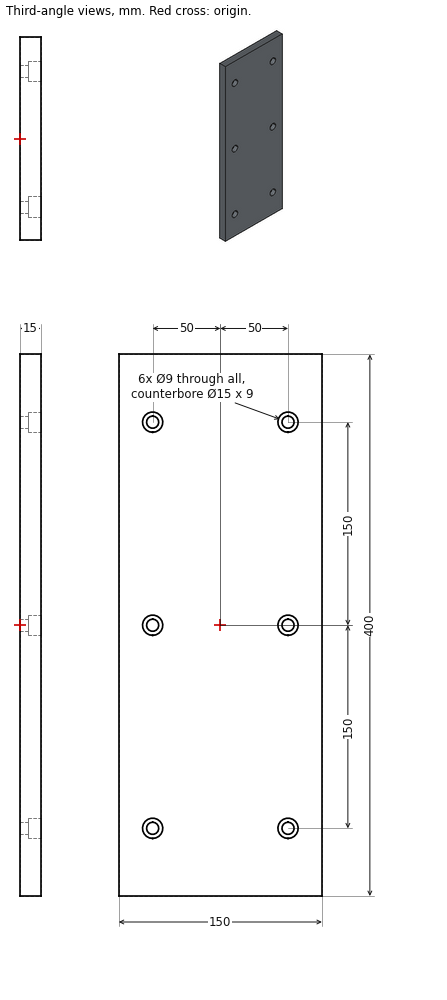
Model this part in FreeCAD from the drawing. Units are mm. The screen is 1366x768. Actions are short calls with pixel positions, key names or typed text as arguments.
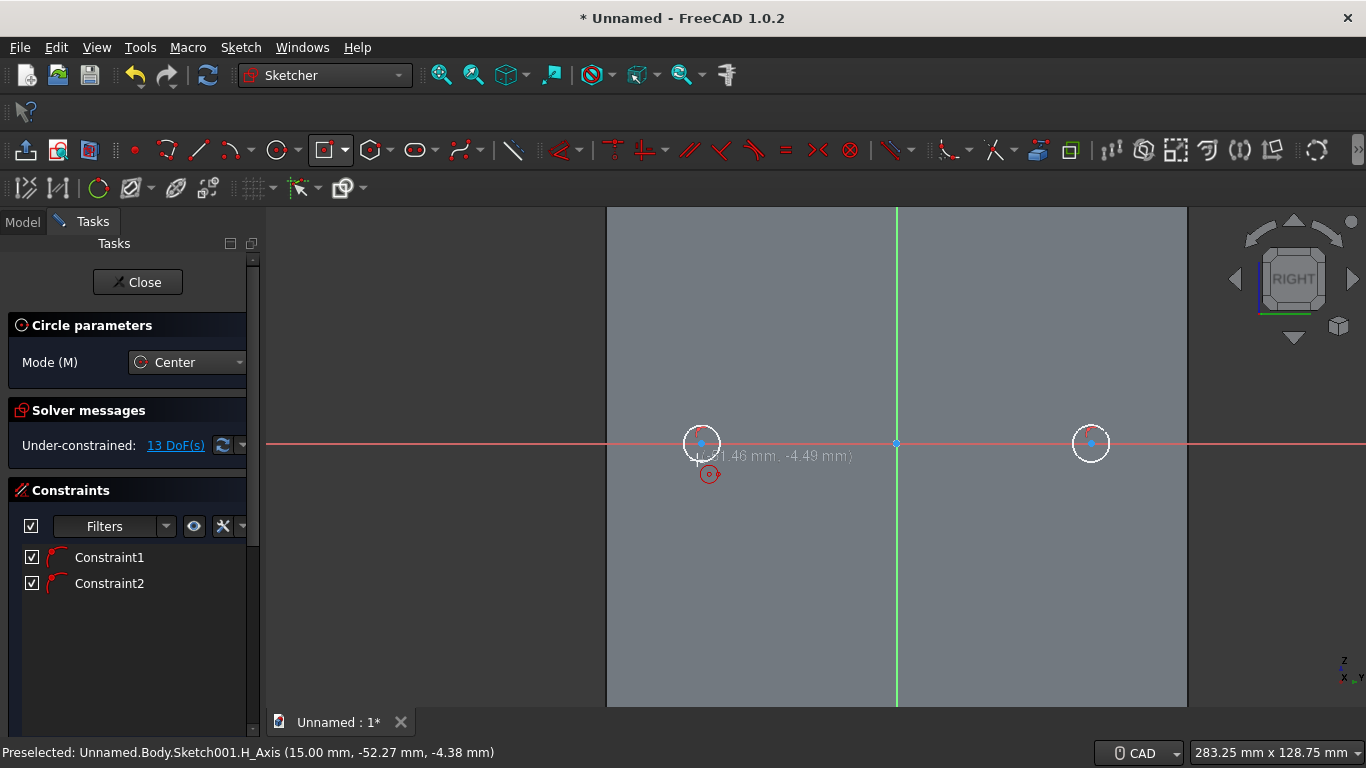
scroll(699, 461, down, 7)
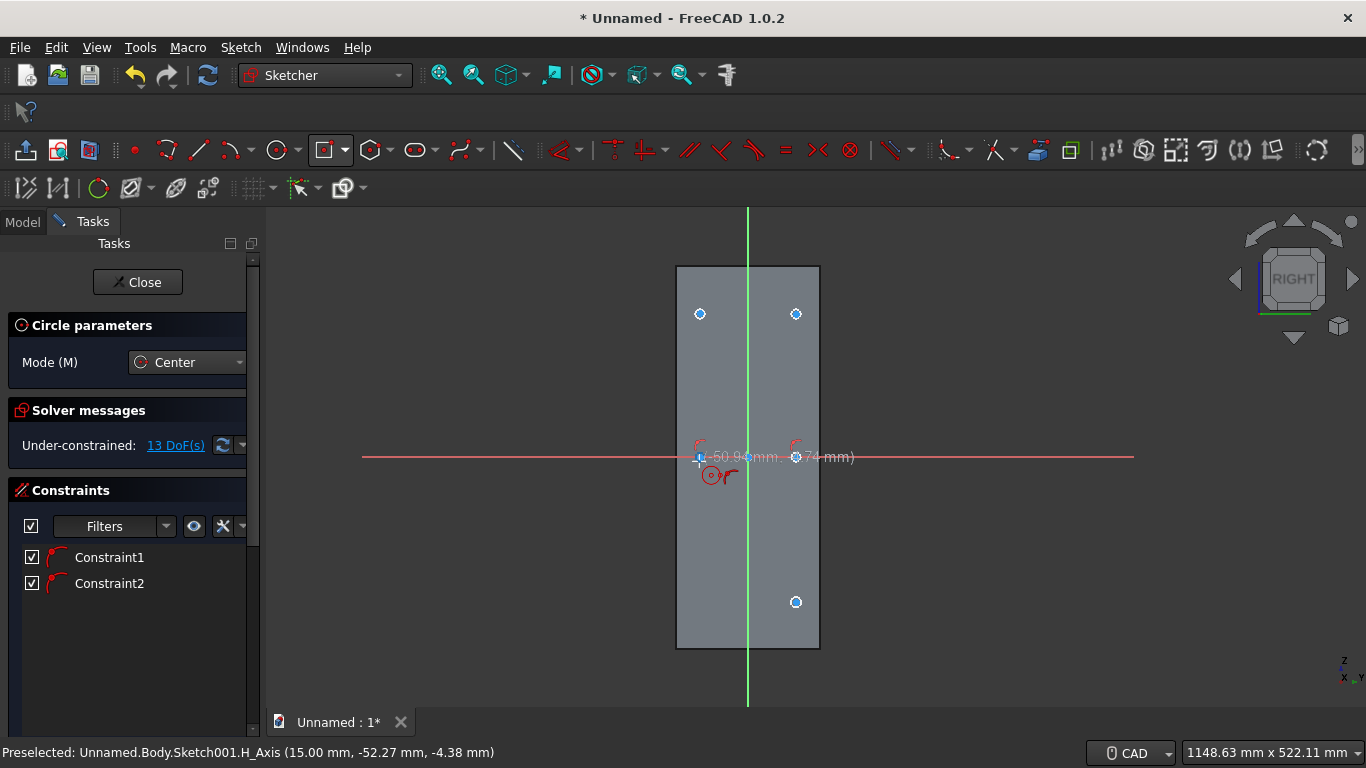
scroll(700, 601, up, 9)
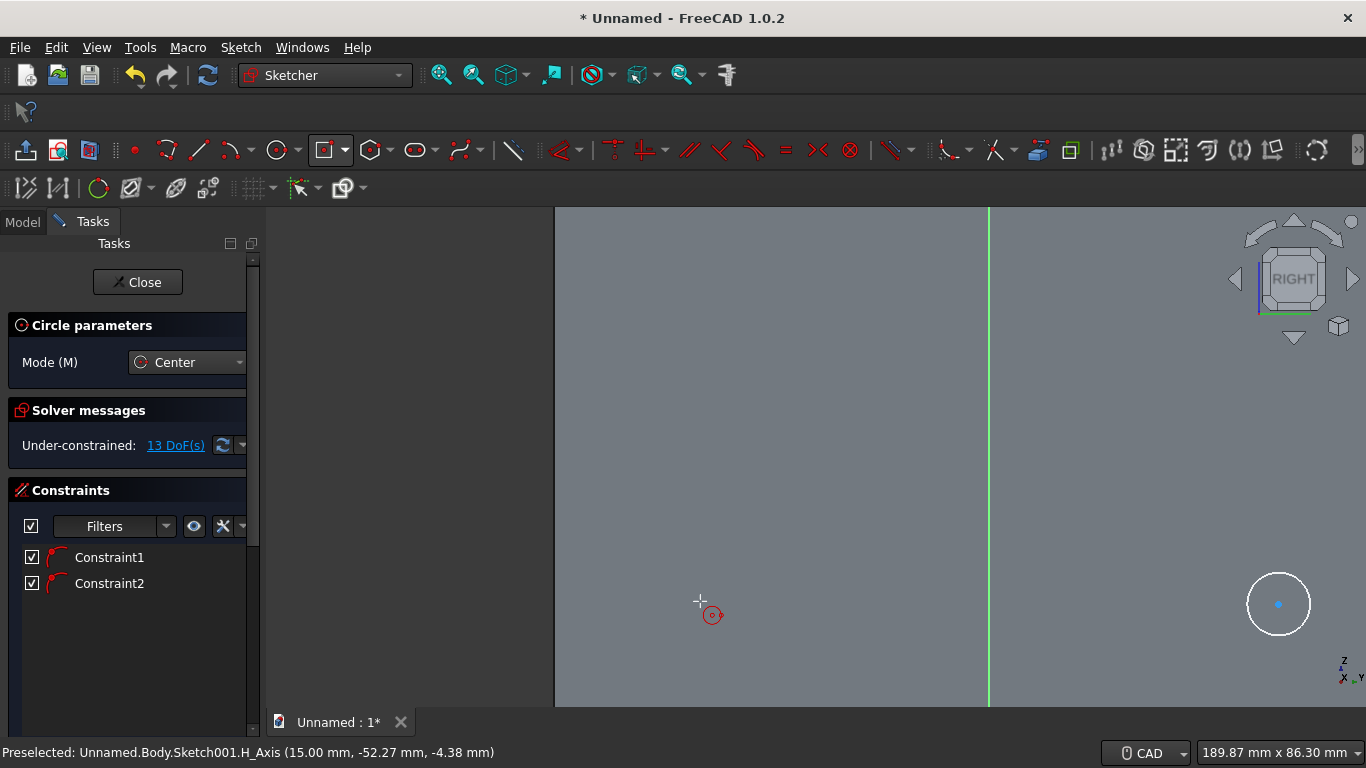
scroll(700, 602, down, 9)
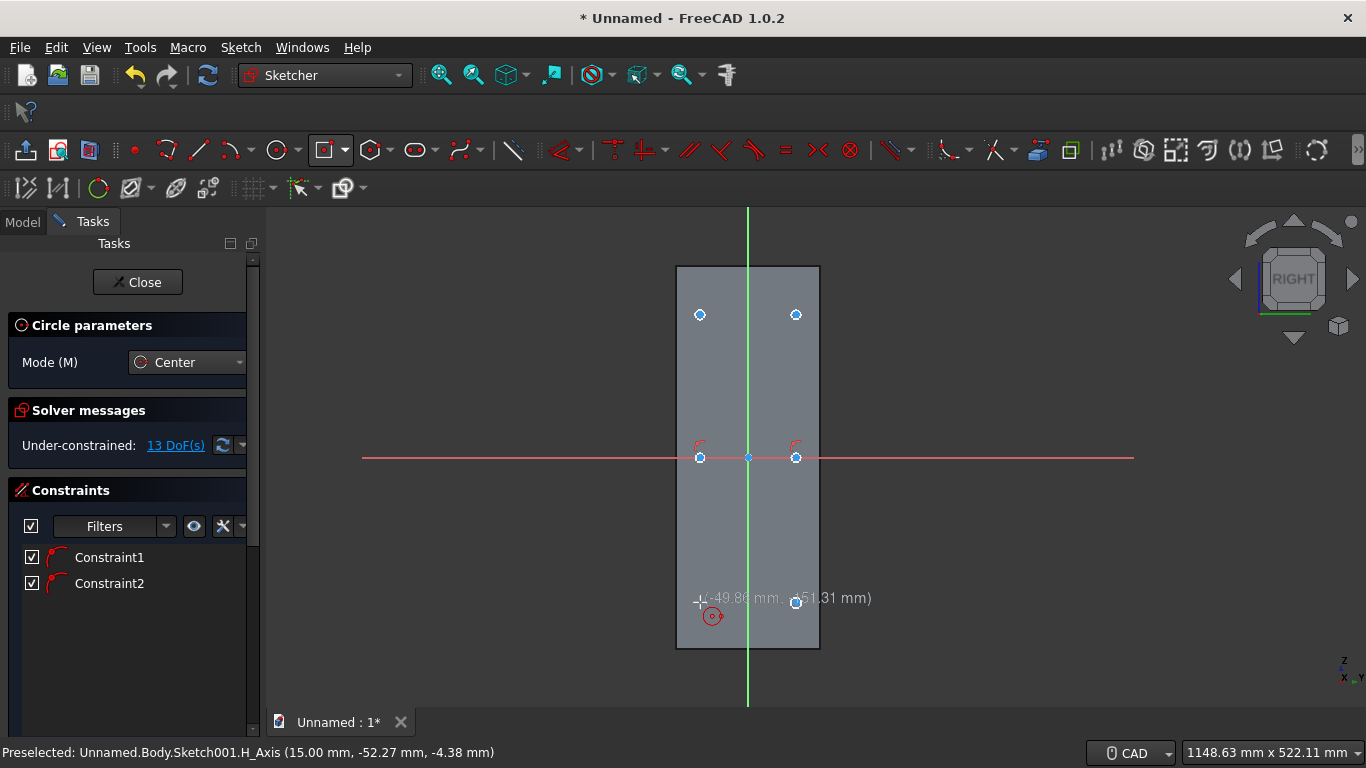
click(700, 602)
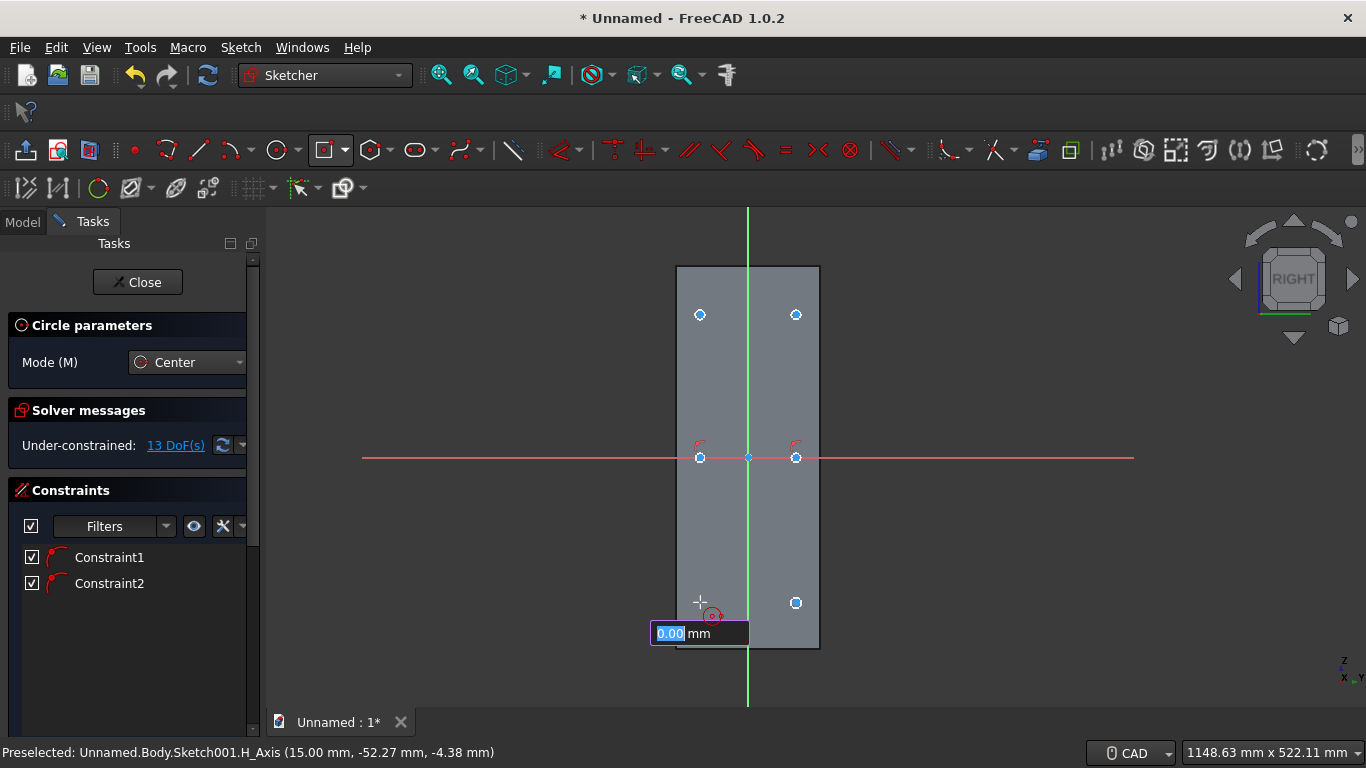
scroll(703, 599, up, 7)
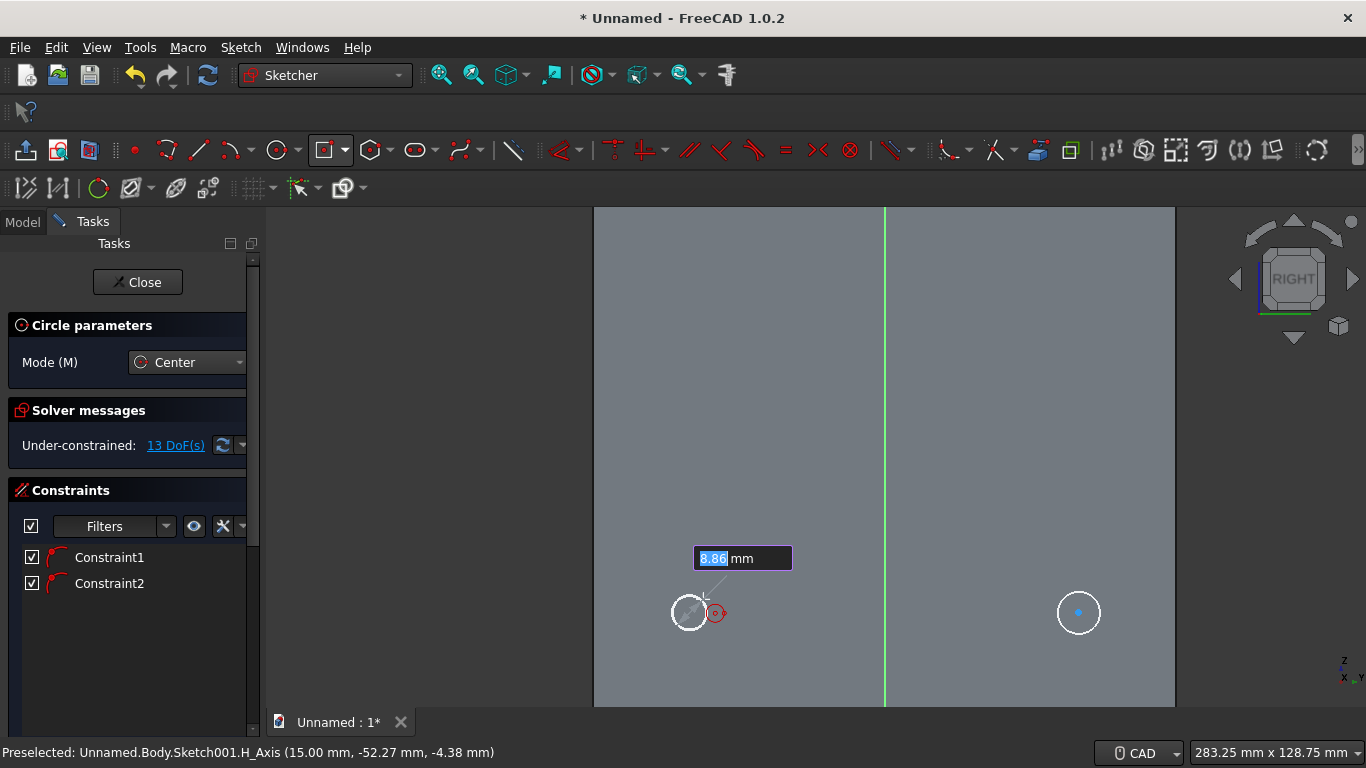
click(703, 595)
key(Escape)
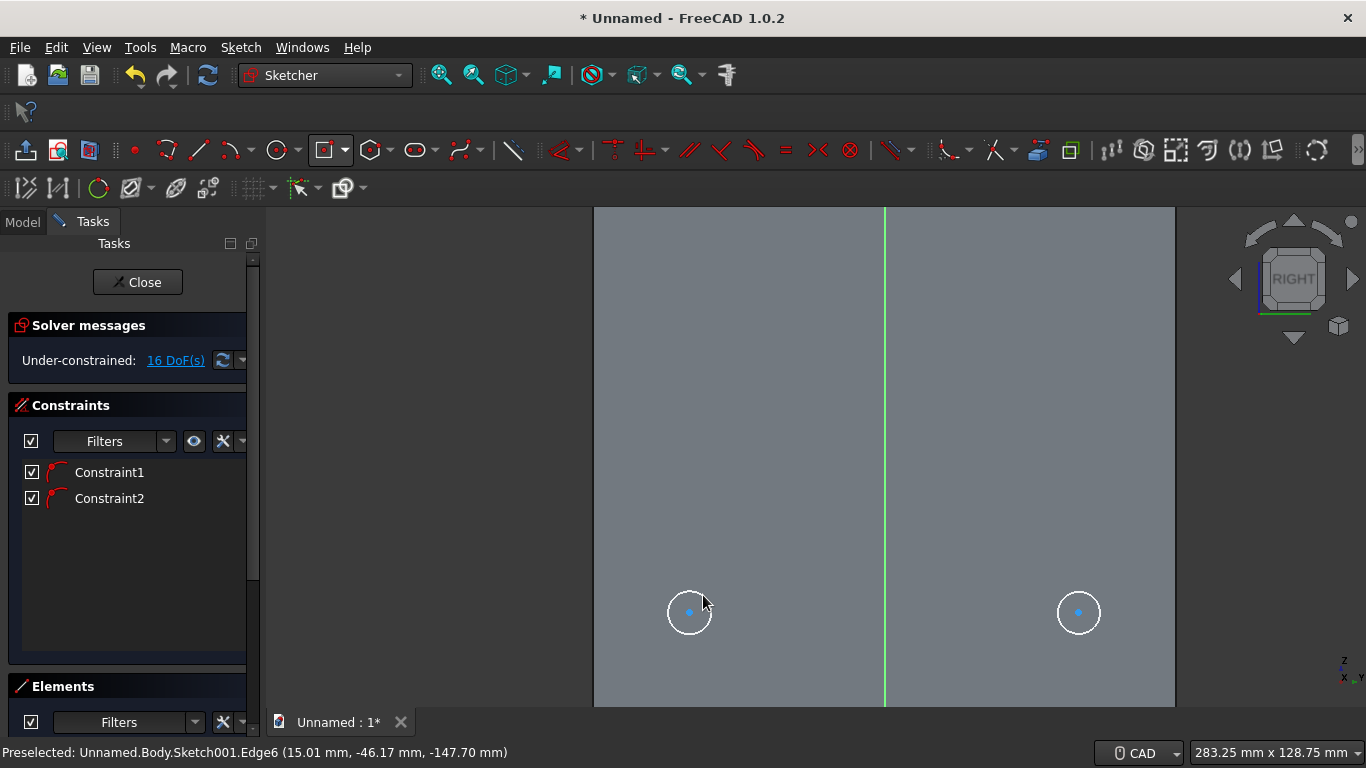
scroll(703, 599, down, 7)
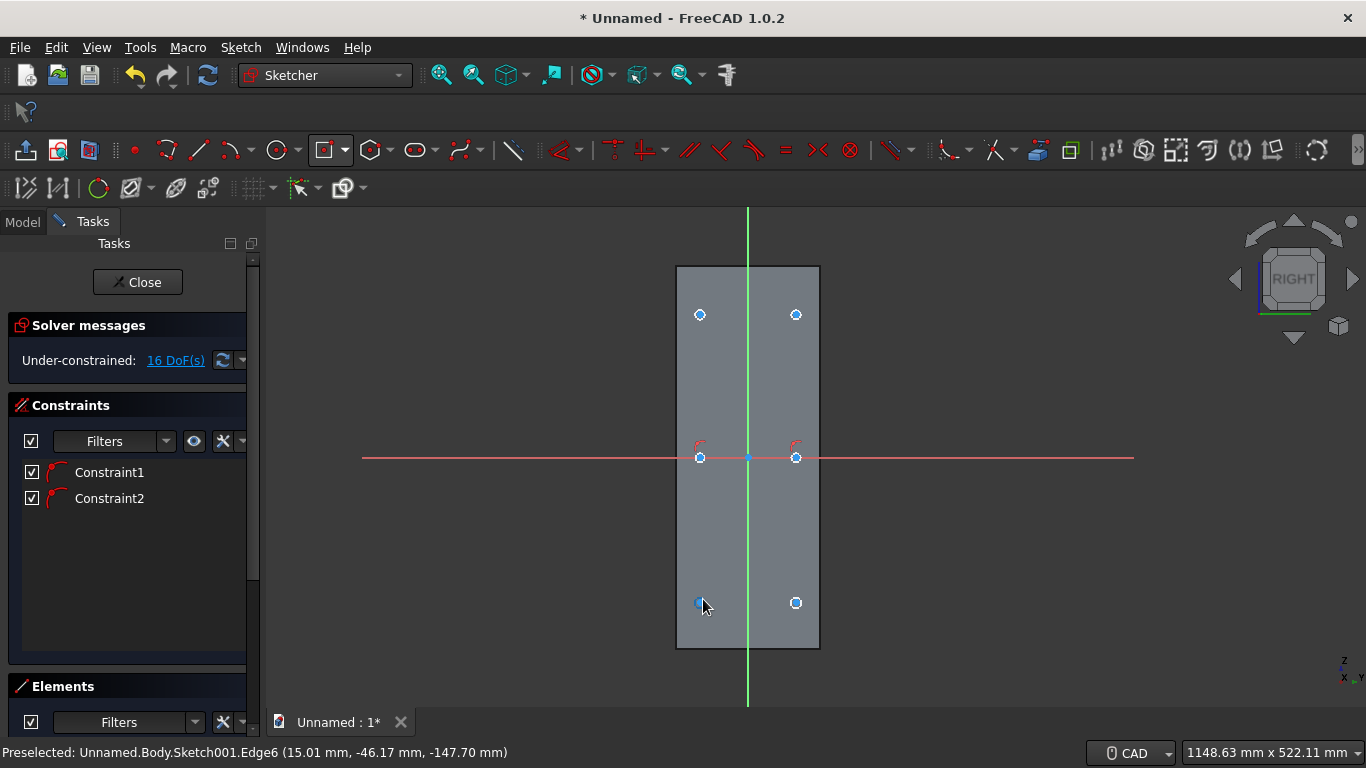
scroll(799, 312, up, 6)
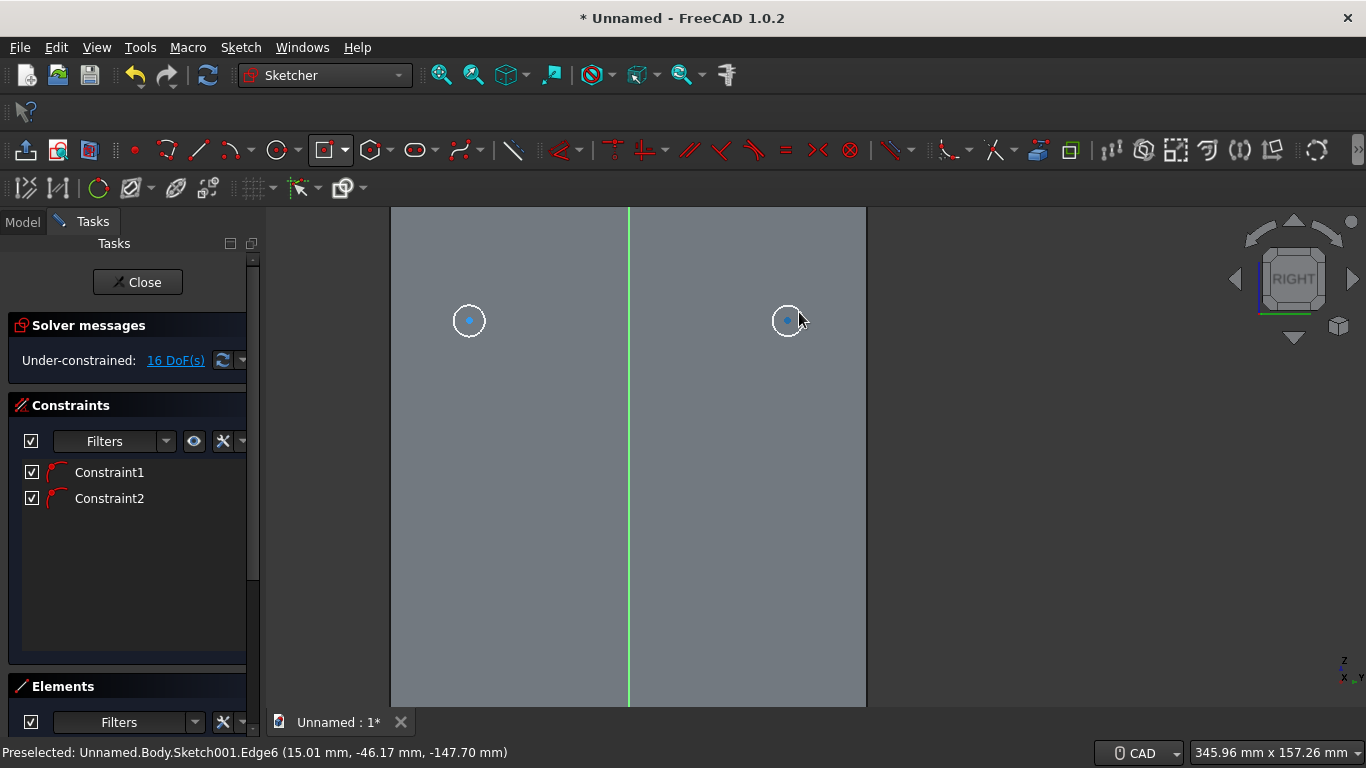
click(799, 310)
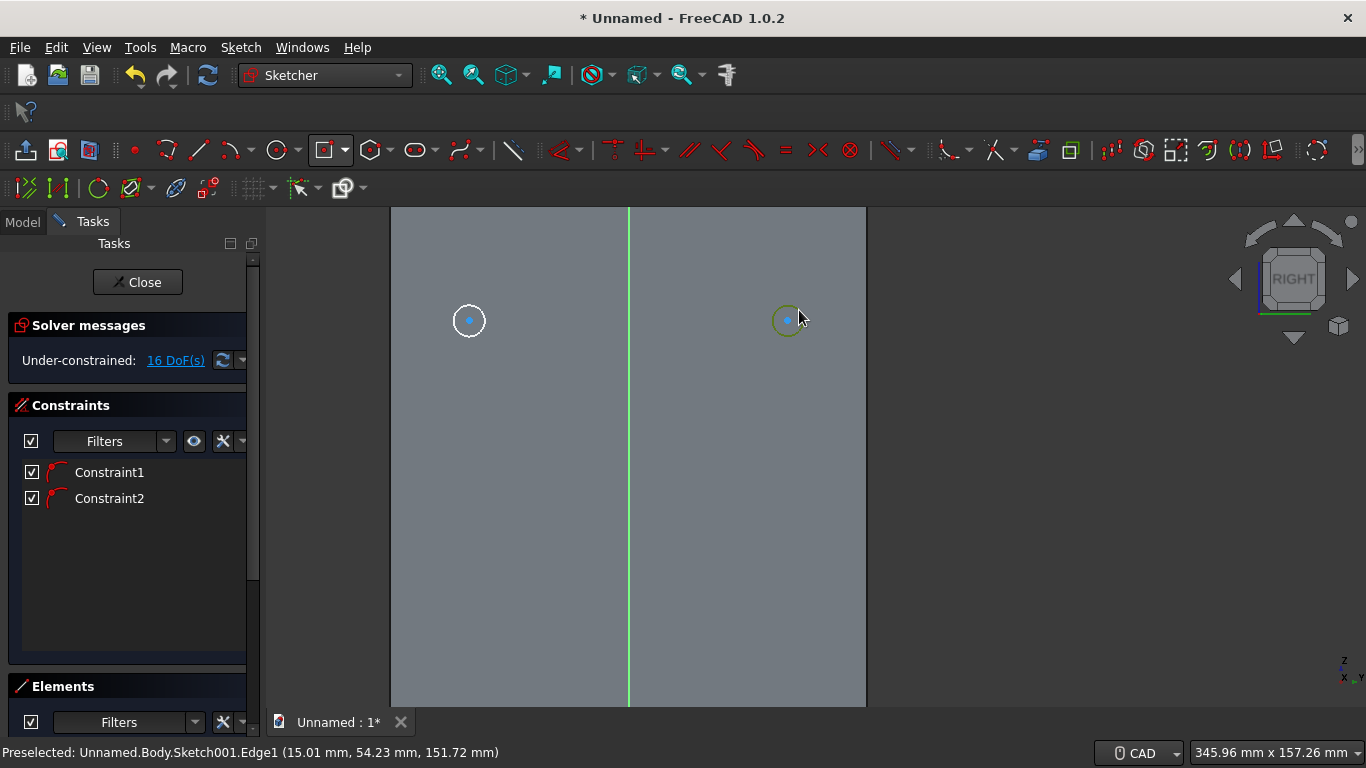
scroll(799, 311, down, 6)